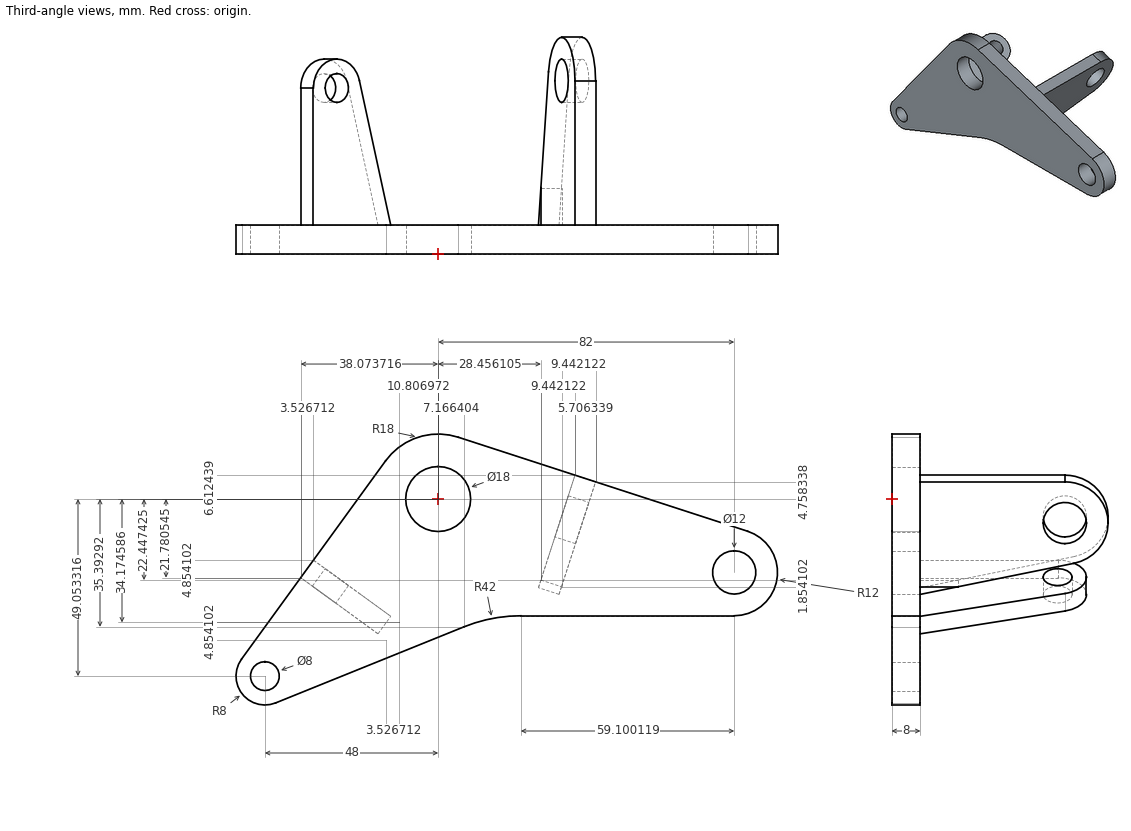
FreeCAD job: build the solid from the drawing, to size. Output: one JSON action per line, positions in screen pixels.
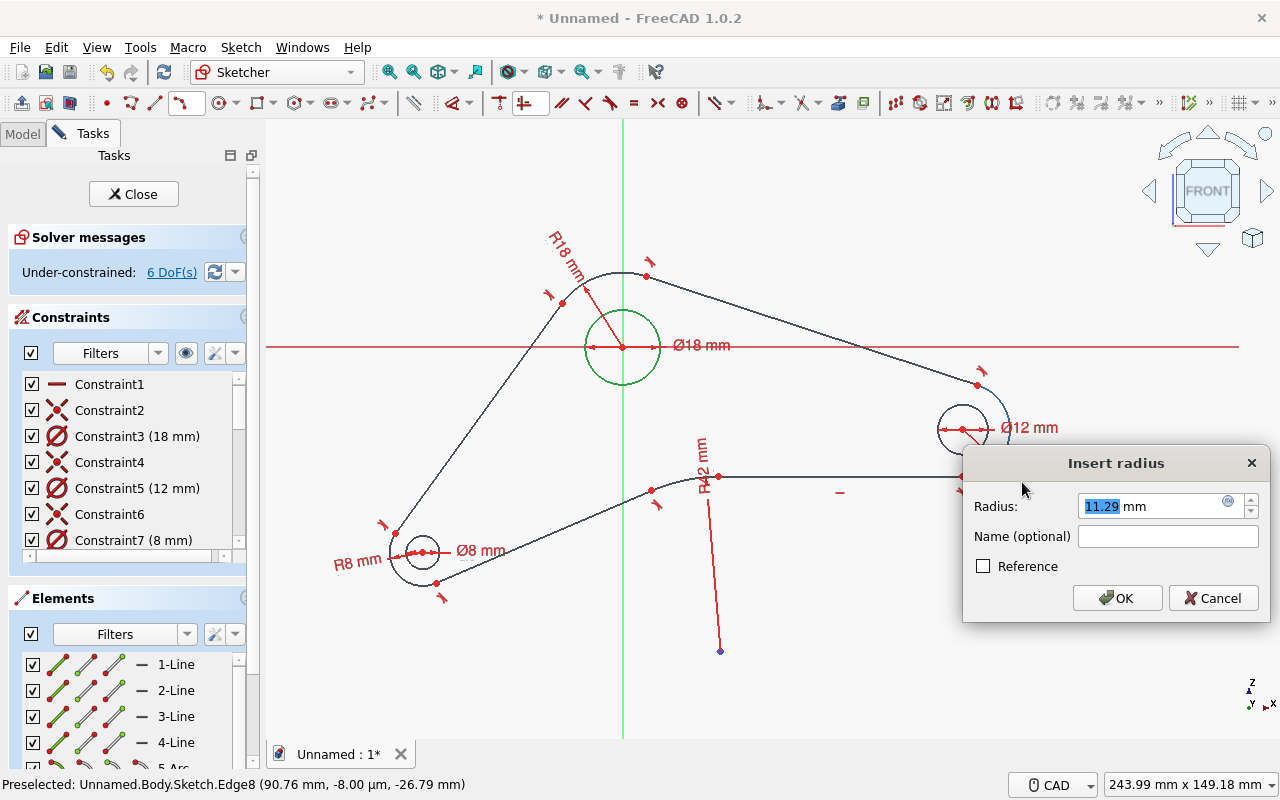
{"action": "type", "text": "12"}
{"action": "key", "text": "Return"}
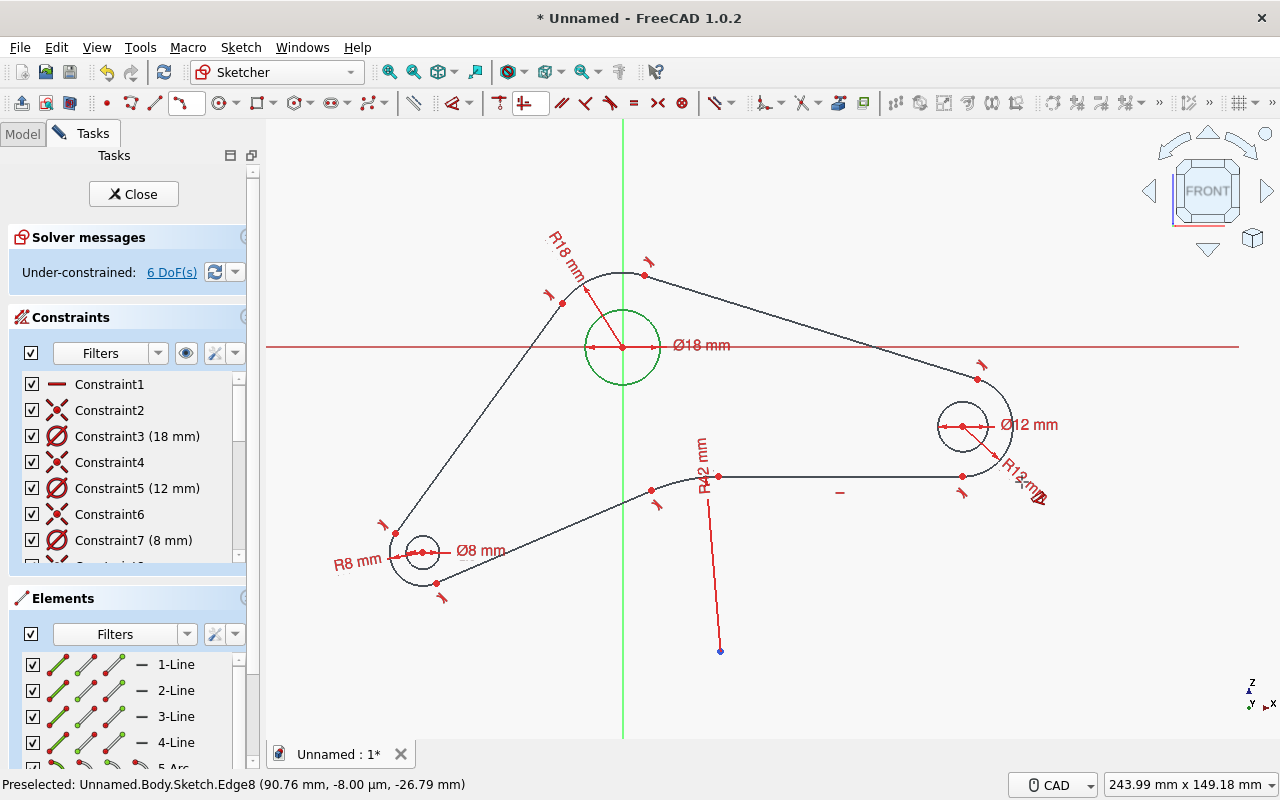
{"action": "left_click", "coordinate": [963, 427]}
{"action": "left_click", "coordinate": [715, 313]}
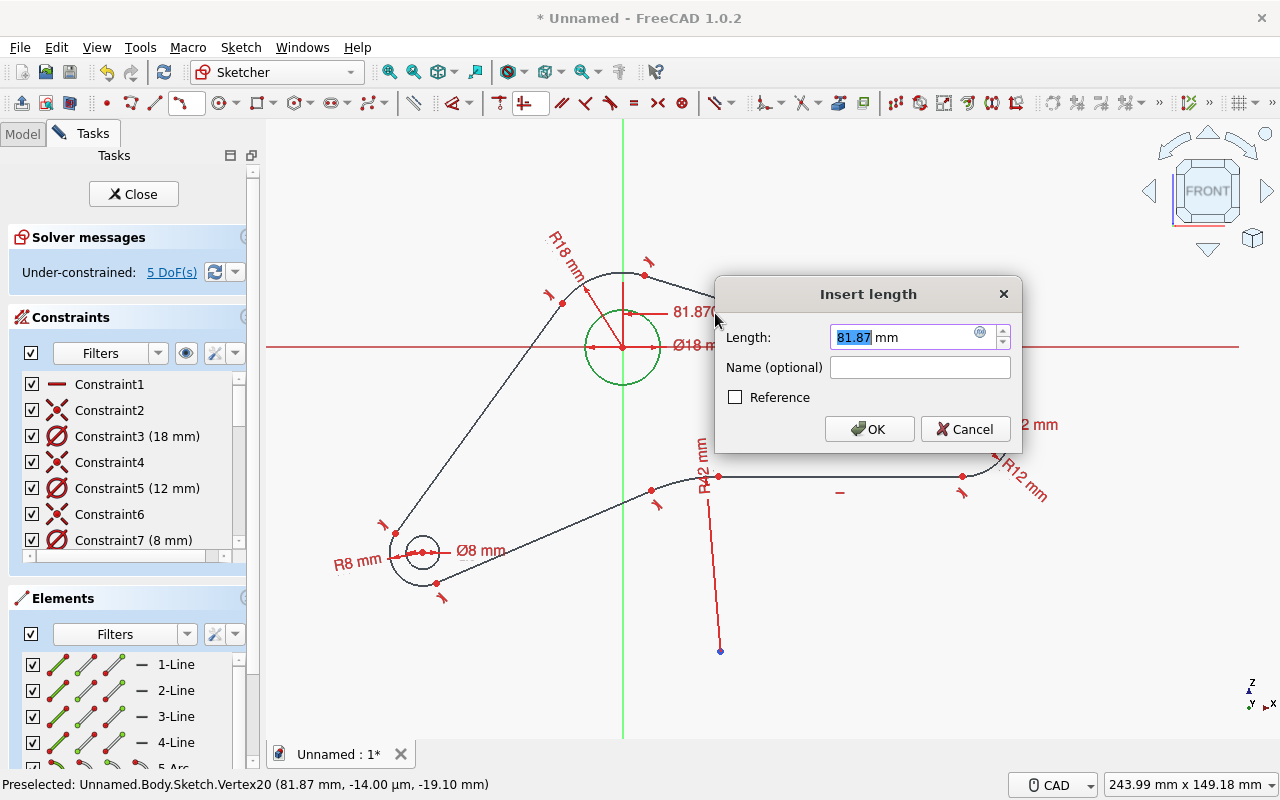
{"action": "type", "text": "82"}
{"action": "key", "text": "Return"}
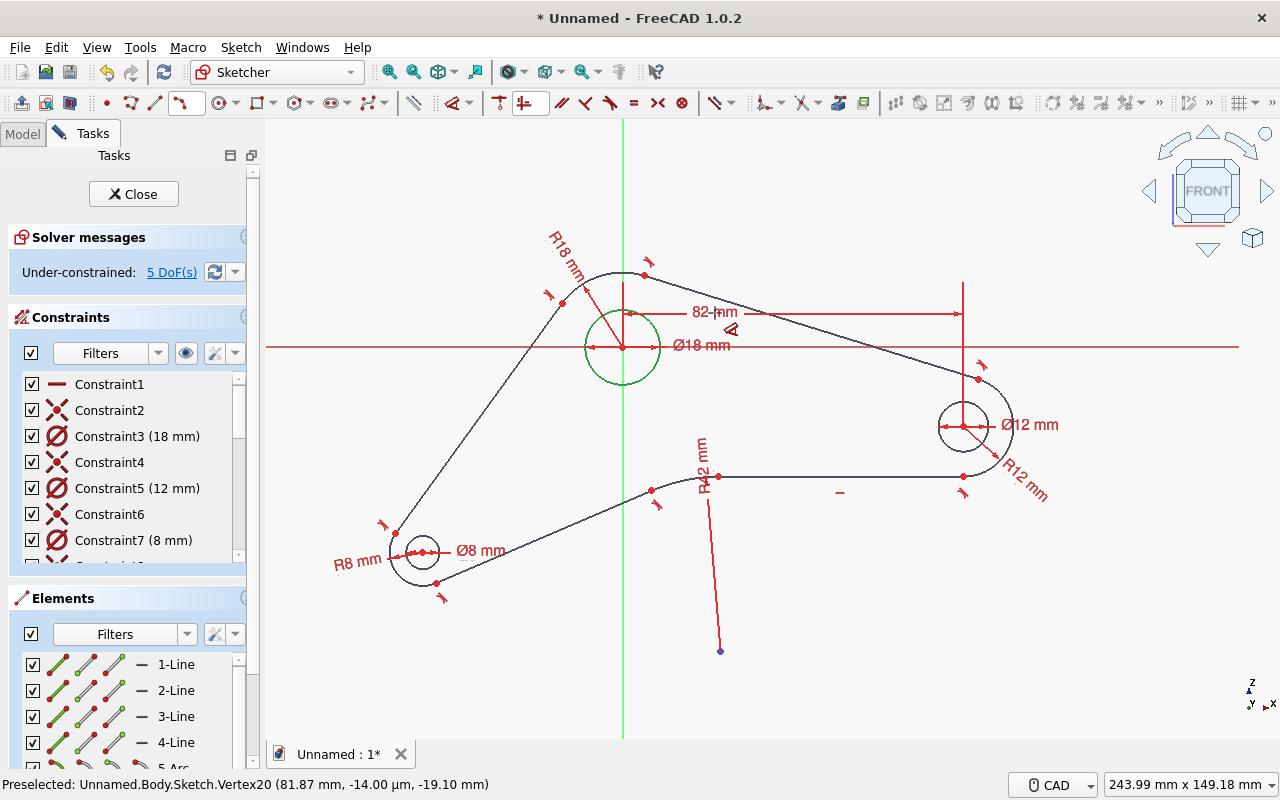
{"action": "left_click", "coordinate": [423, 553]}
{"action": "left_click", "coordinate": [523, 587]}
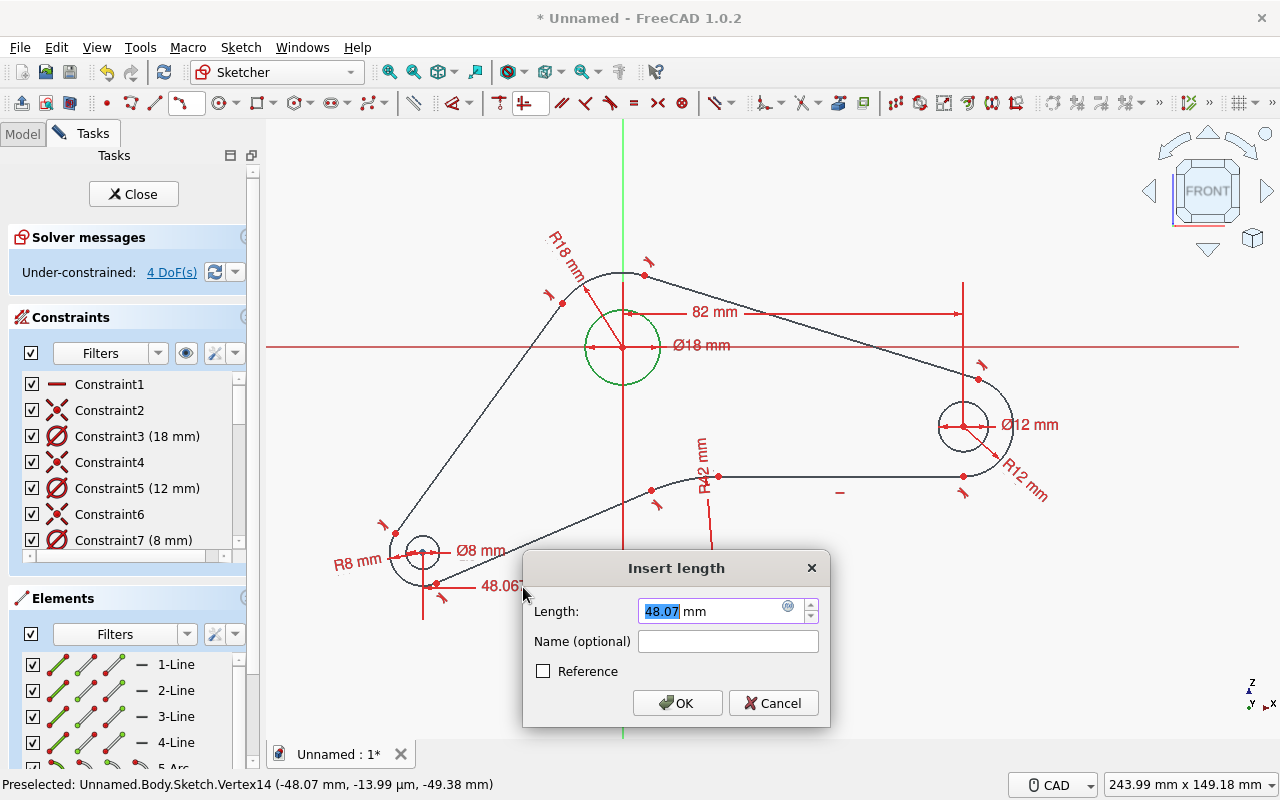
{"action": "type", "text": "48"}
{"action": "key", "text": "Return"}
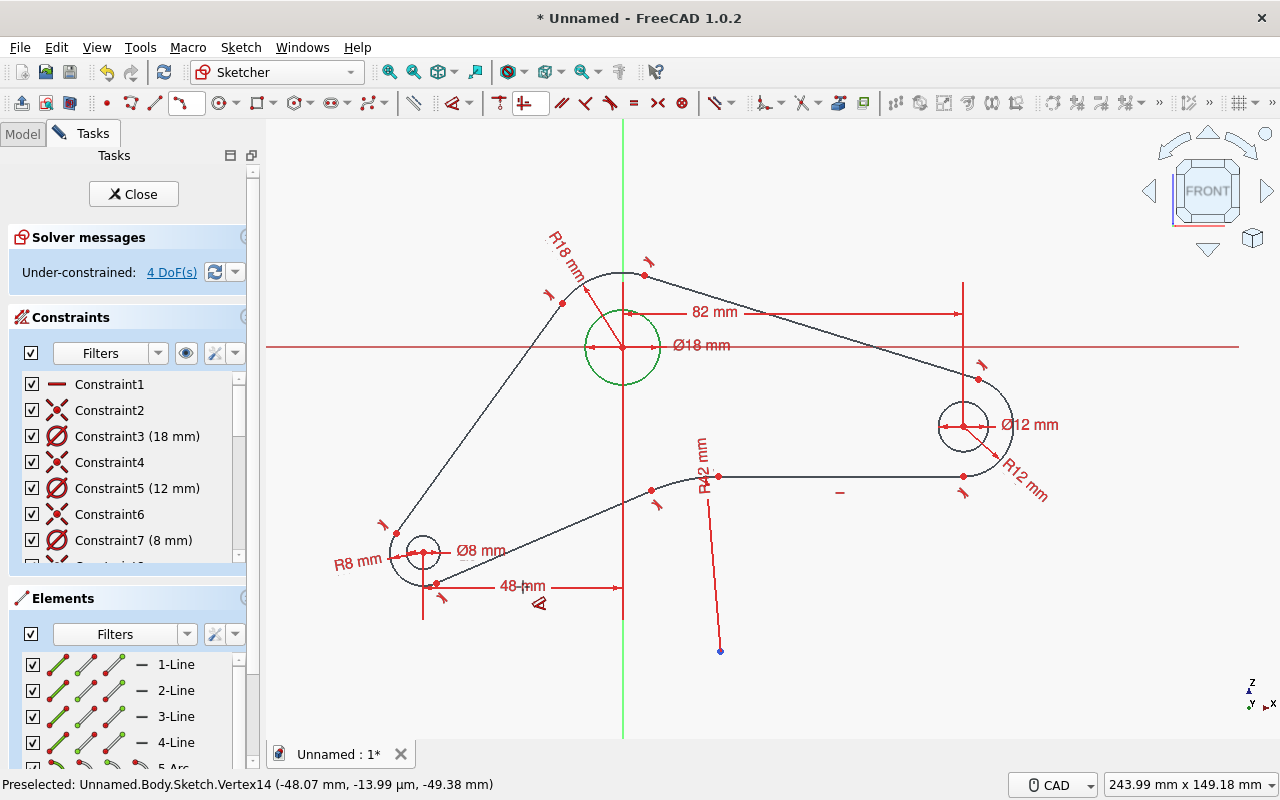
{"action": "left_click", "coordinate": [890, 477]}
{"action": "left_click", "coordinate": [841, 511]}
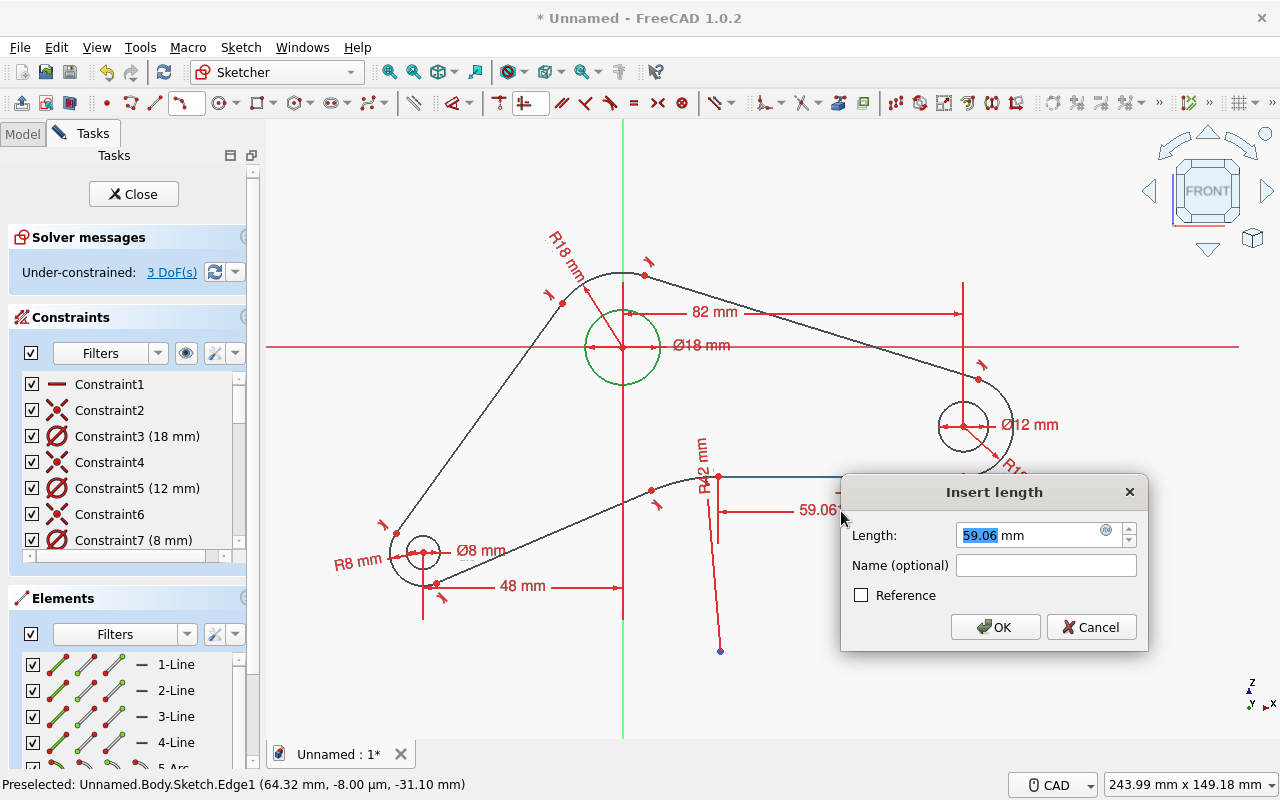
{"action": "type", "text": "59.100119"}
{"action": "key", "text": "Return"}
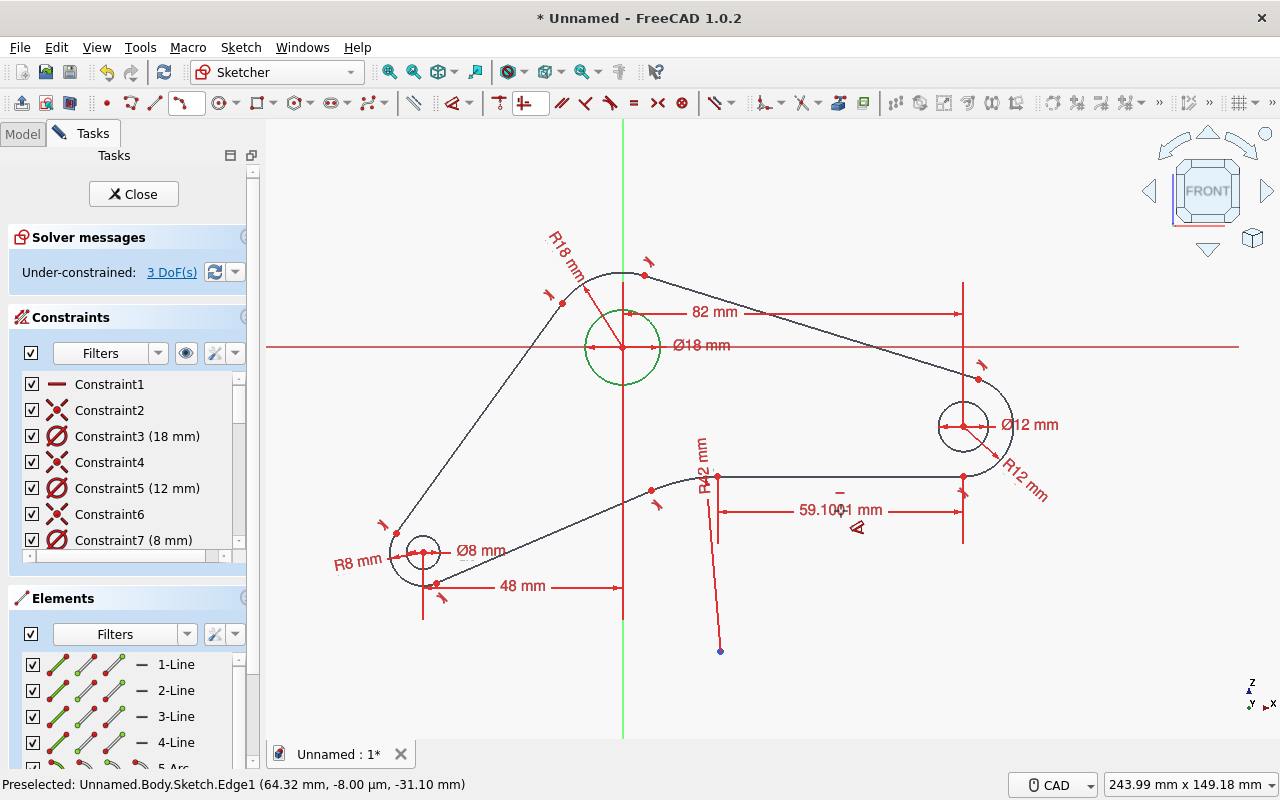
{"action": "scroll", "coordinate": [652, 491], "scroll_direction": "up", "scroll_amount": 2}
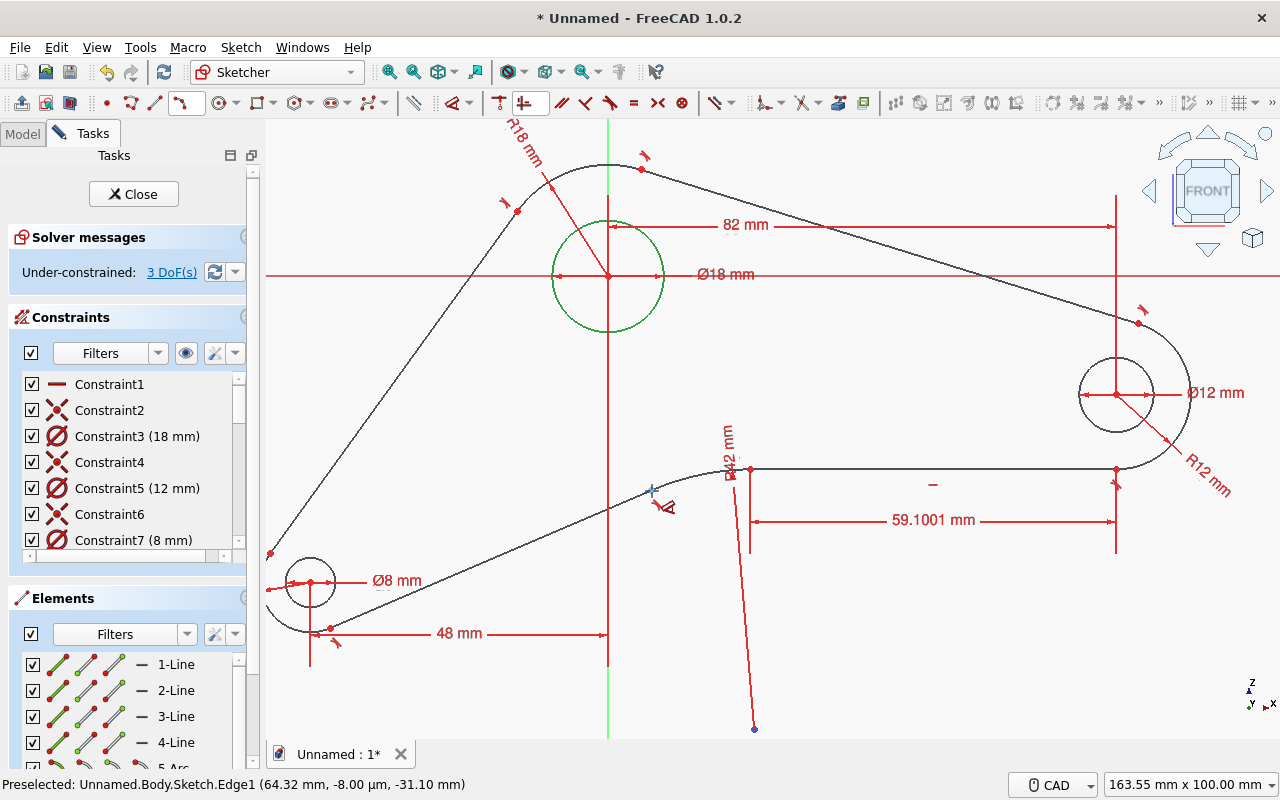
{"action": "left_click", "coordinate": [652, 490]}
{"action": "left_click", "coordinate": [630, 242]}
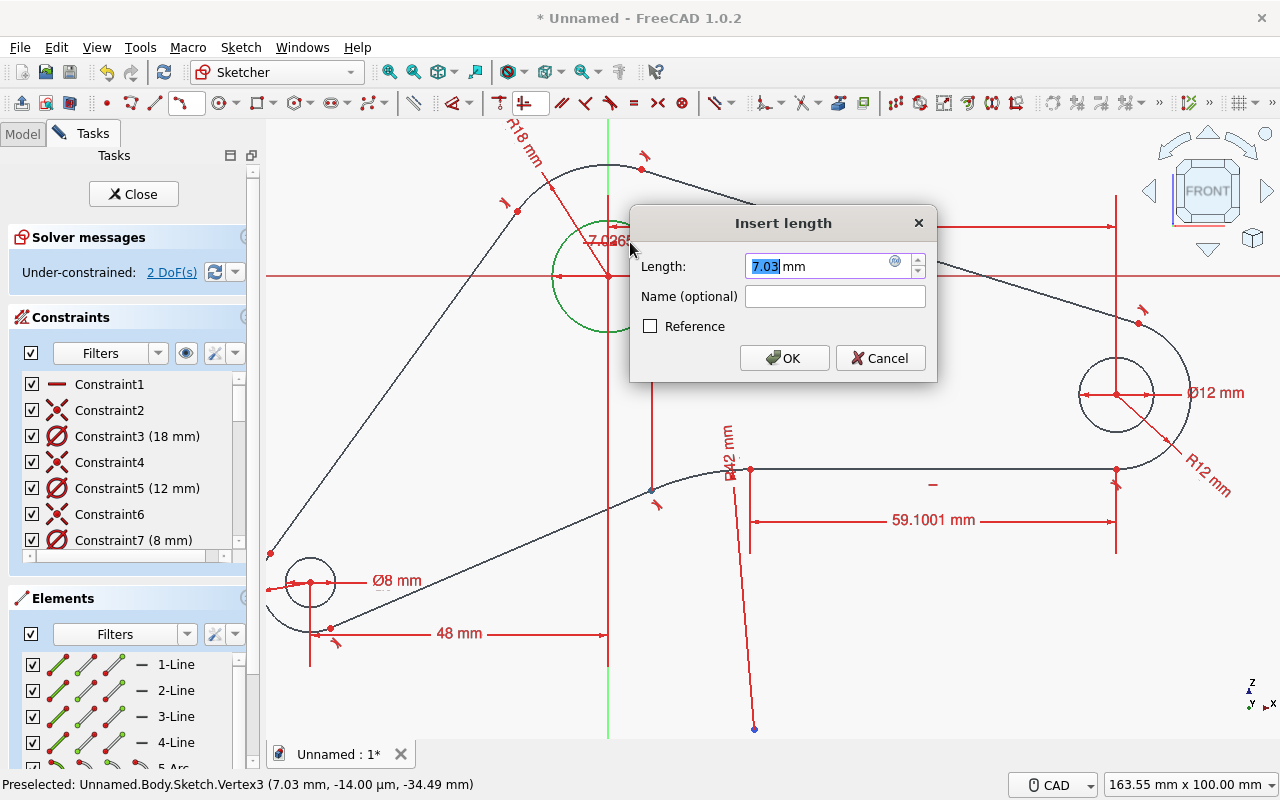
{"action": "type", "text": "7.166404"}
{"action": "key", "text": "Return"}